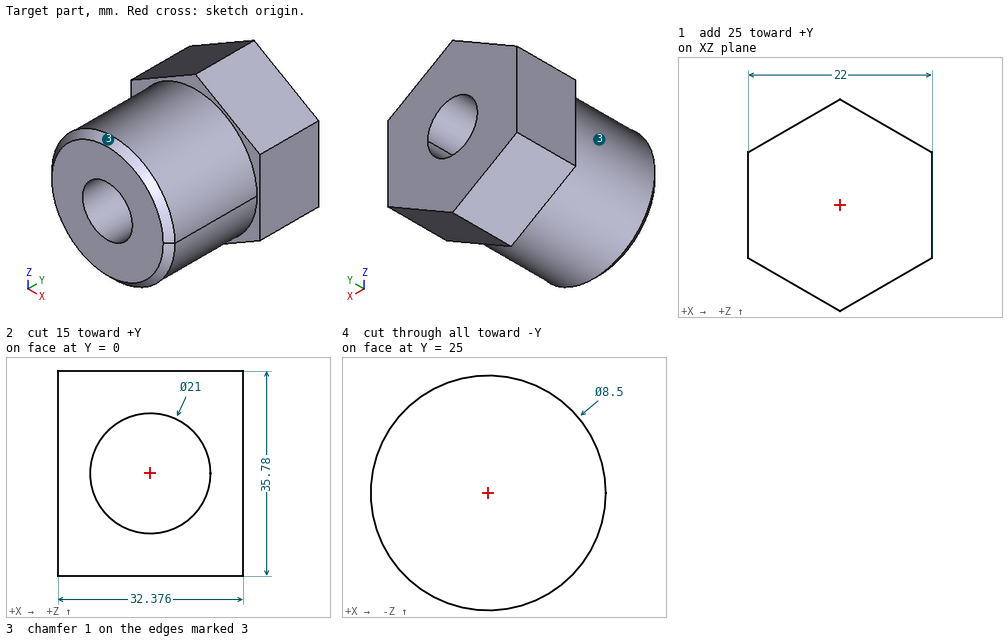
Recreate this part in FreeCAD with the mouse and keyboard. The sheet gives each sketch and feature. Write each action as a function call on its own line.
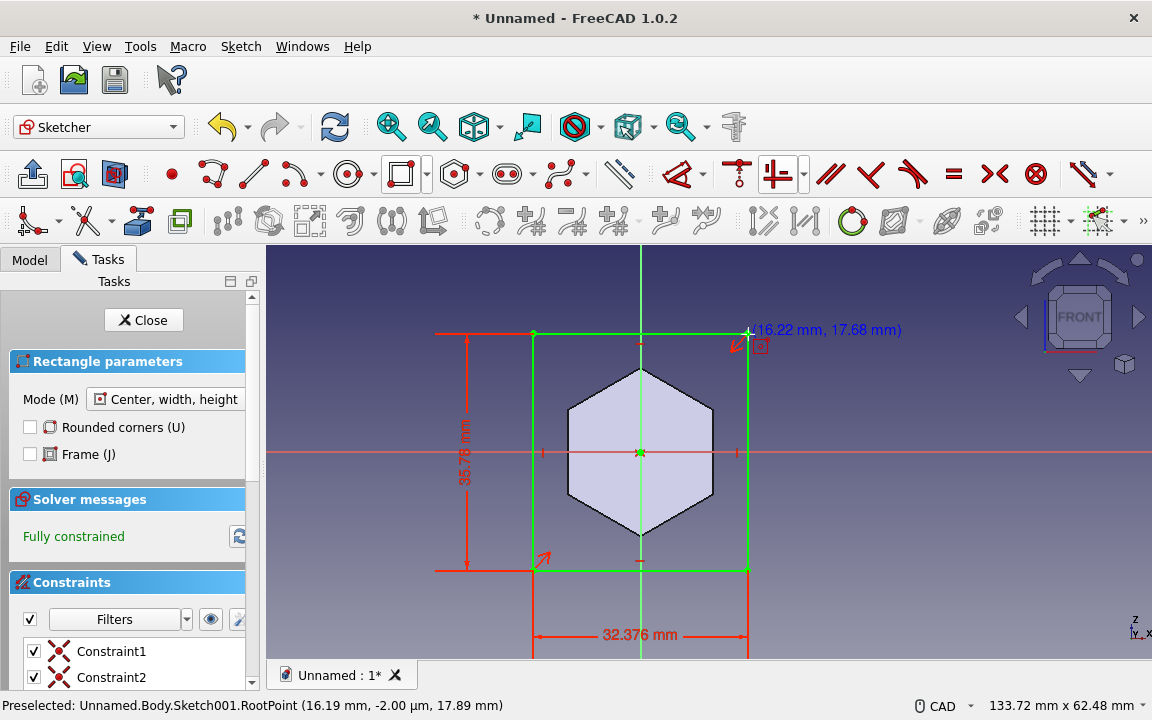
key(g)
key(c)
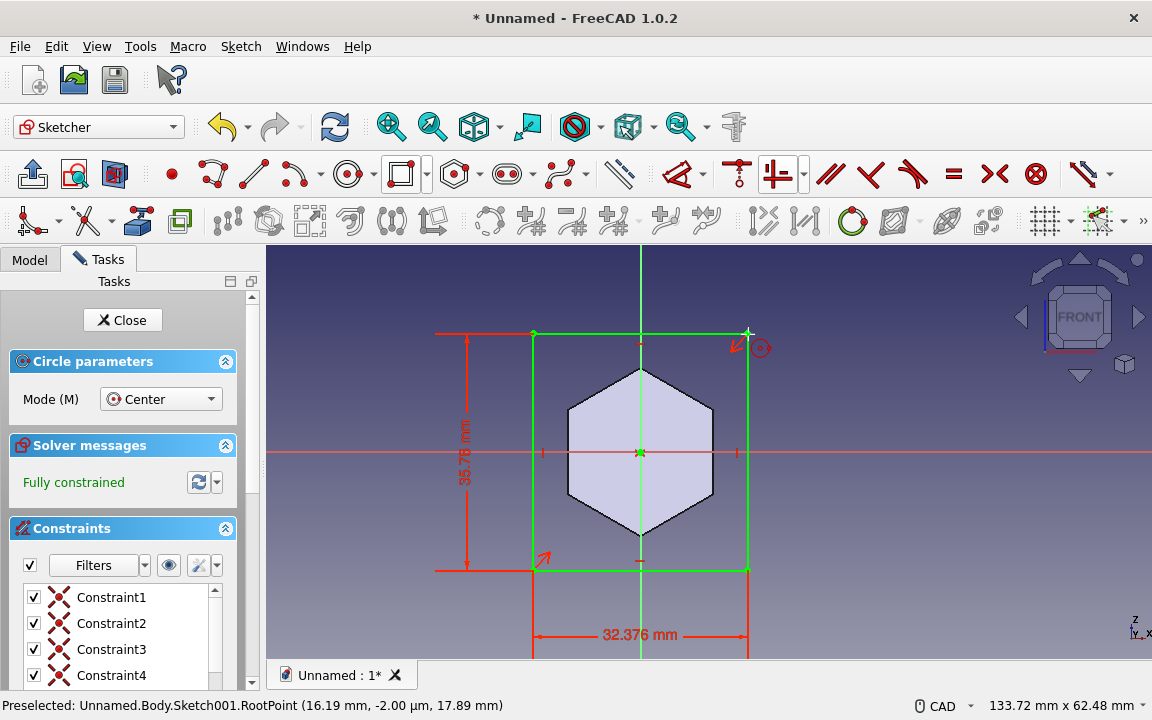
click(641, 452)
move(690, 403)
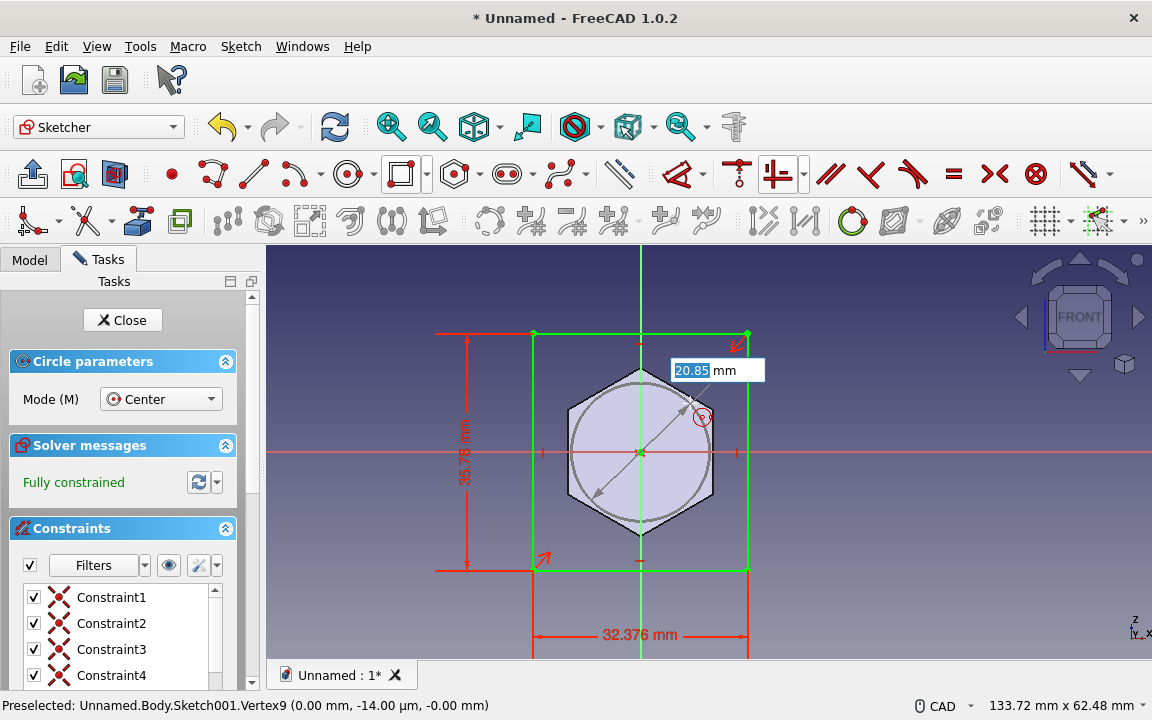
text(21)
key(Return)
key(Escape)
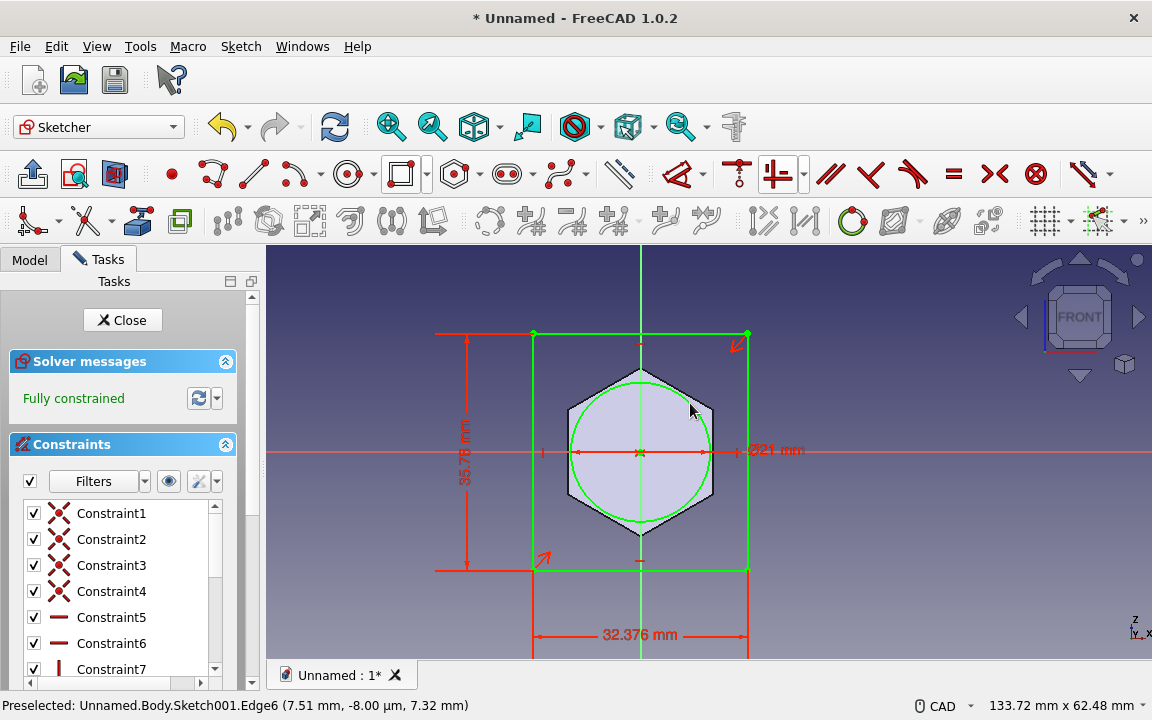
click(123, 320)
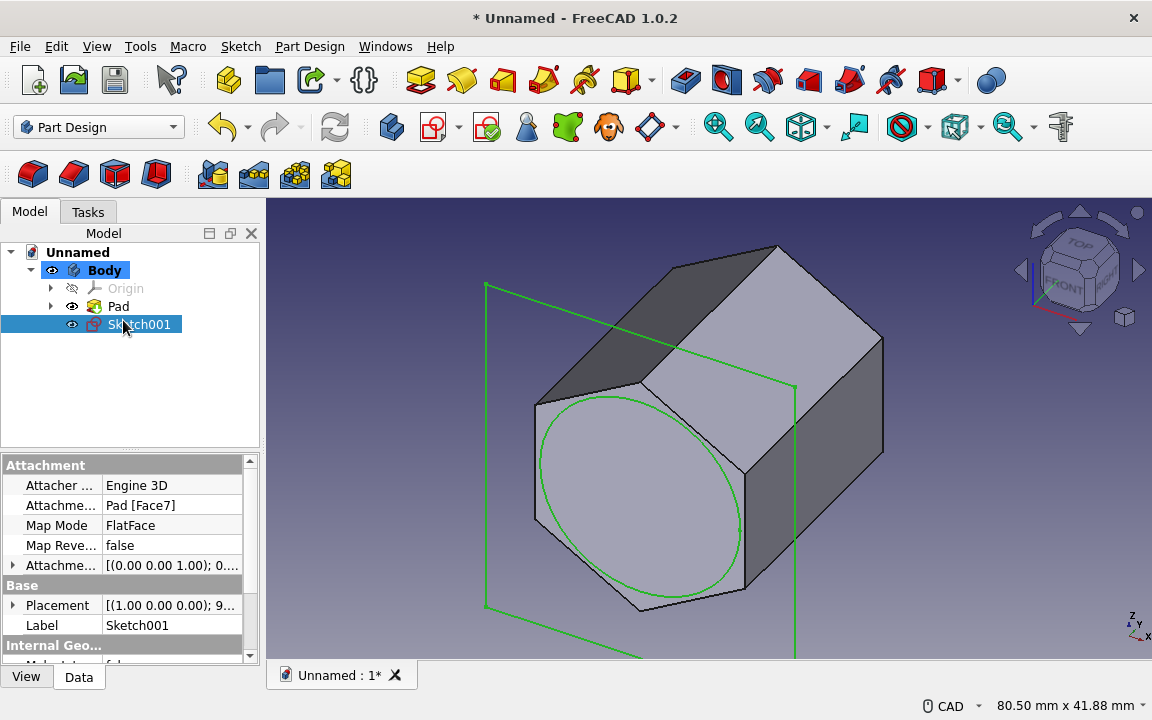
click(686, 80)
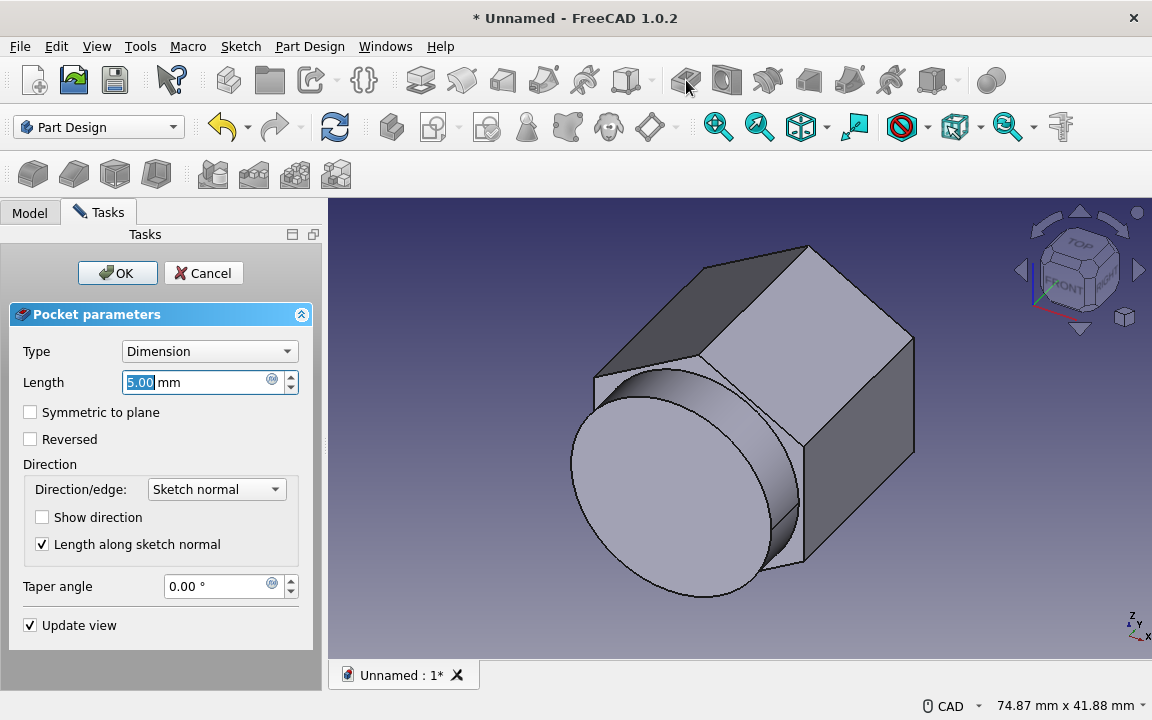
text(15)
key(Tab)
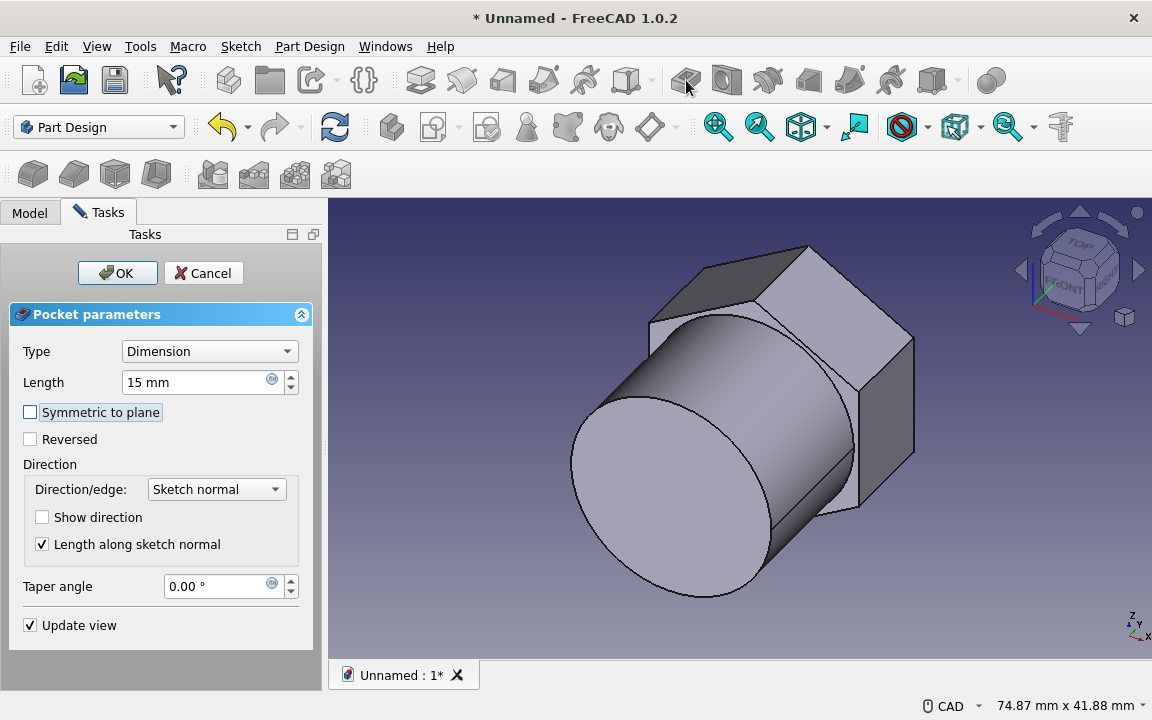
click(118, 273)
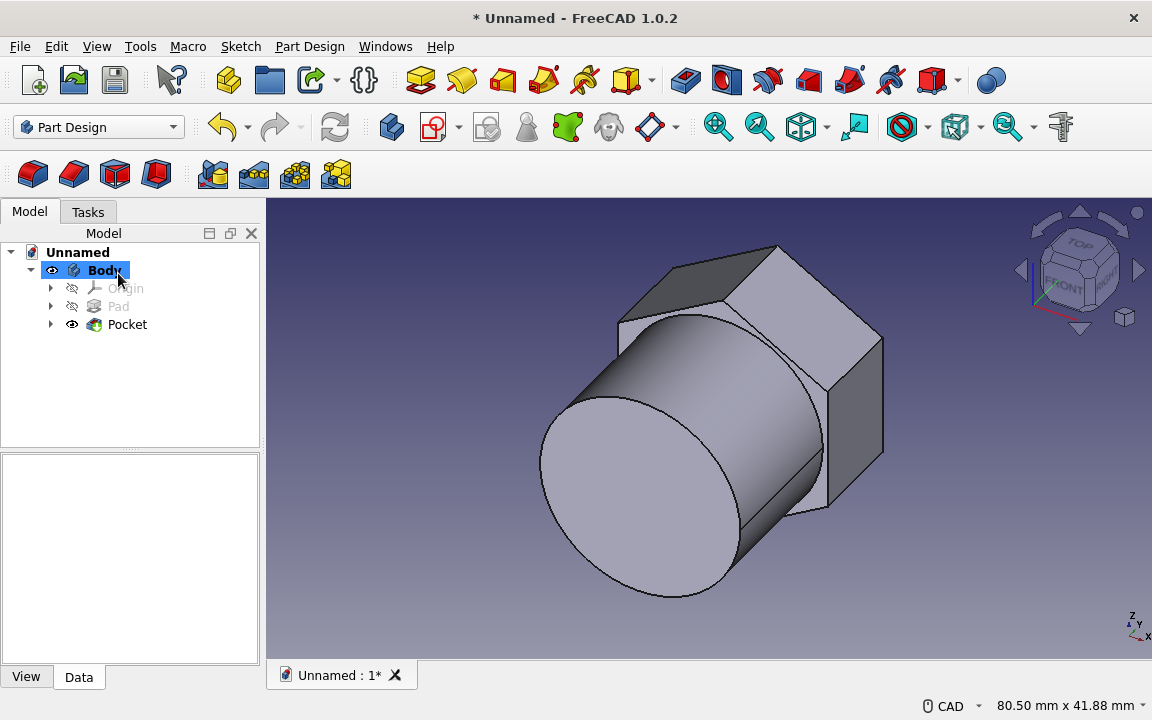
click(559, 413)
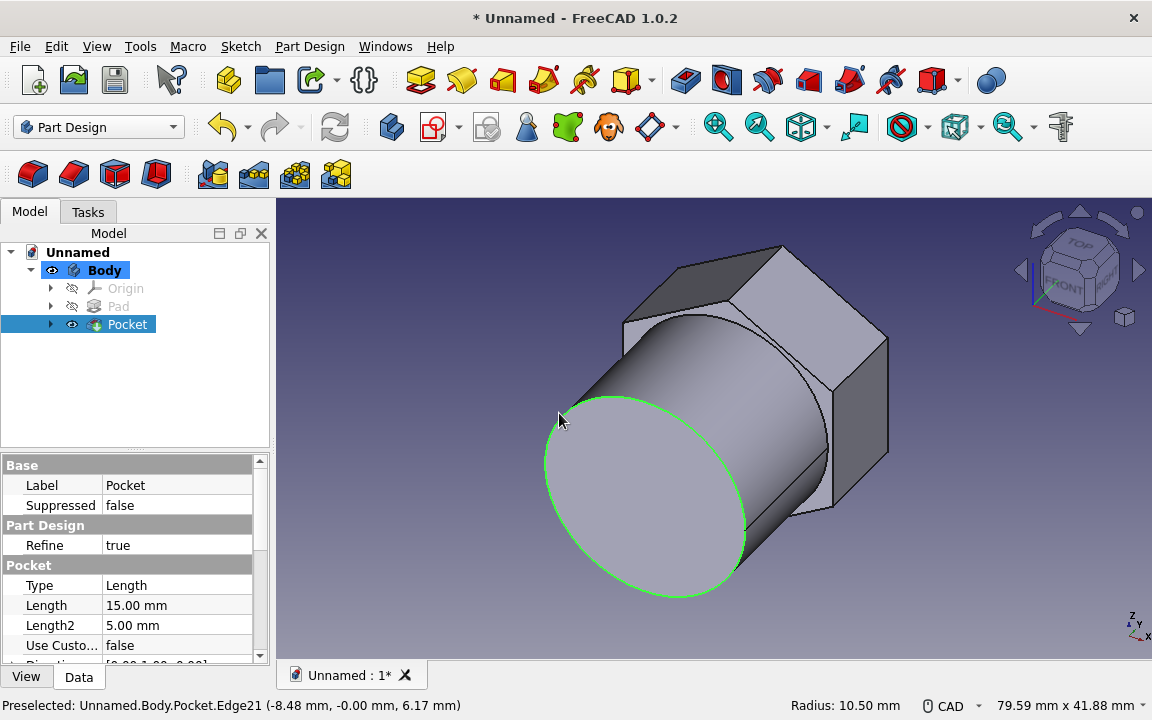
click(74, 174)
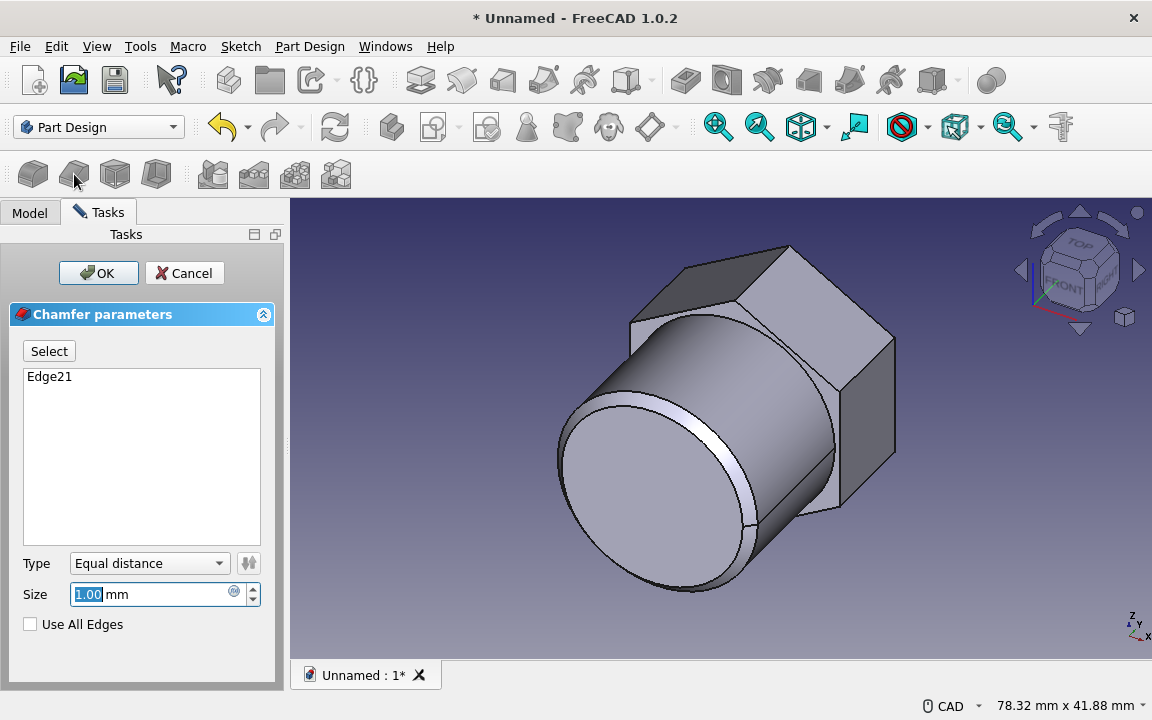
text(1)
key(Tab)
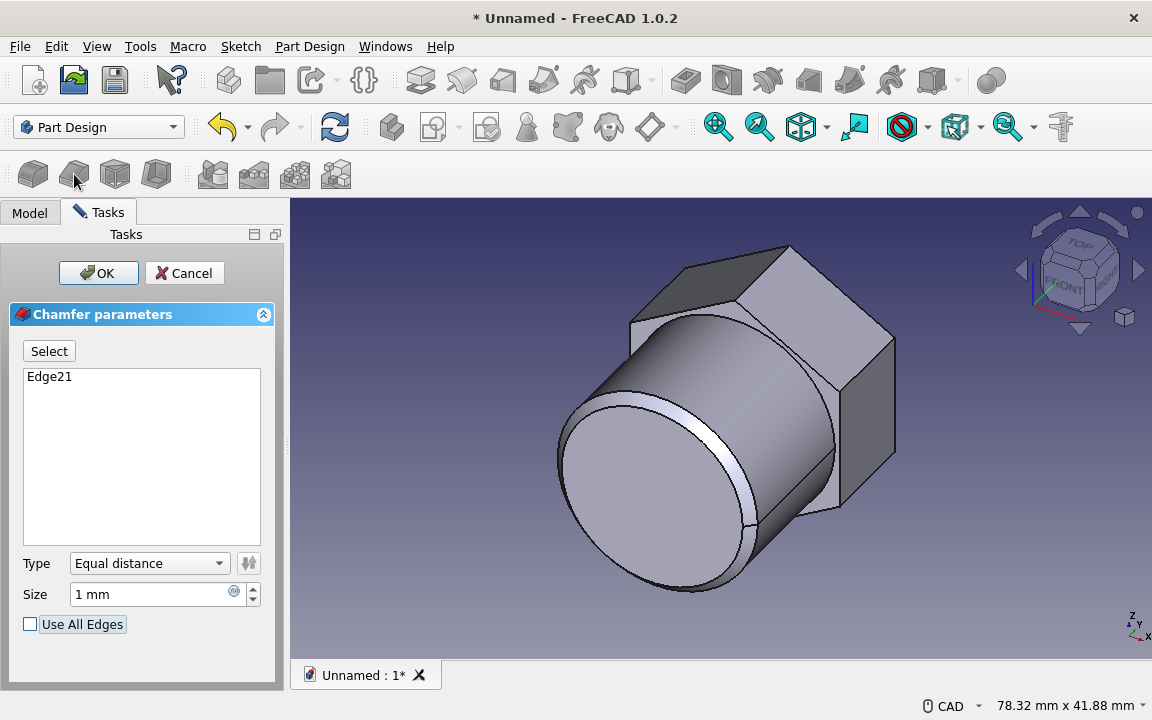
click(99, 273)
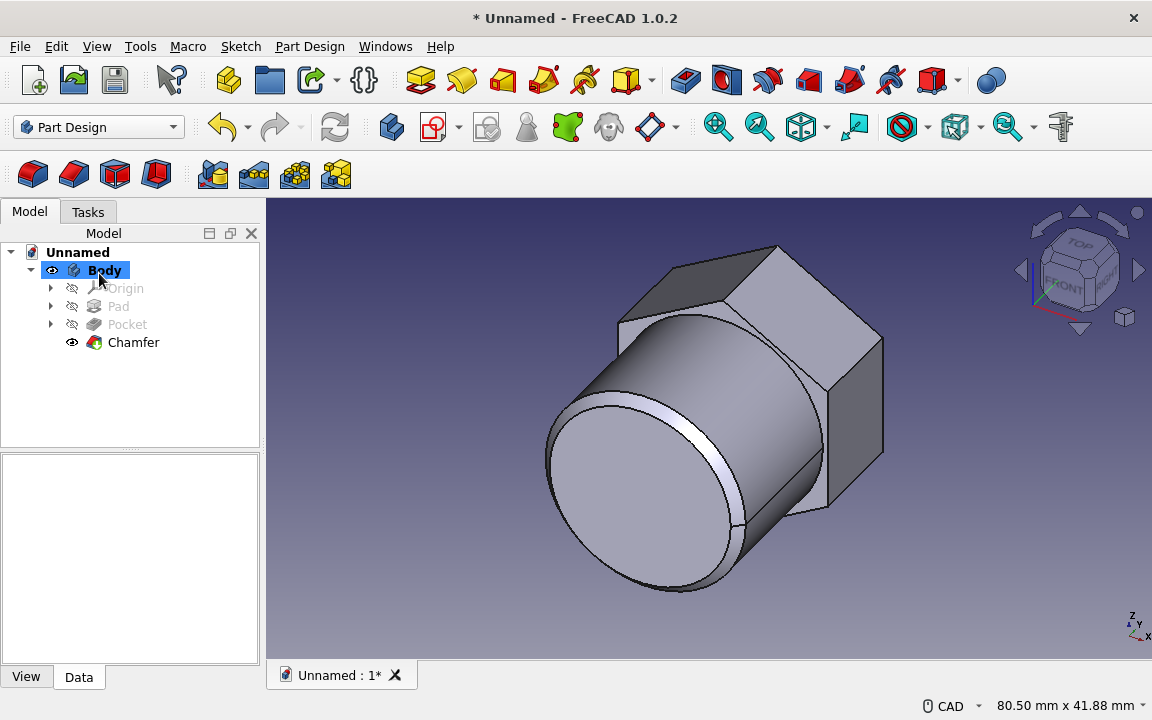
key(4)